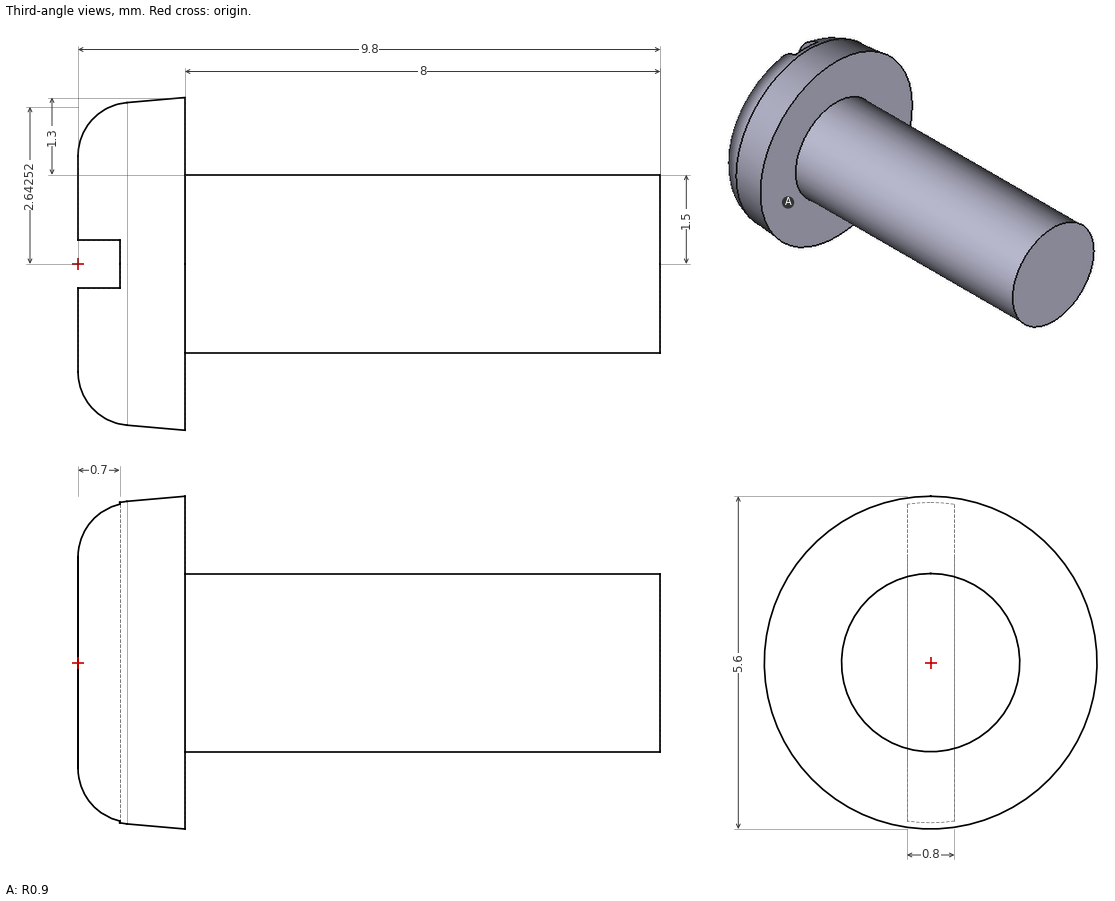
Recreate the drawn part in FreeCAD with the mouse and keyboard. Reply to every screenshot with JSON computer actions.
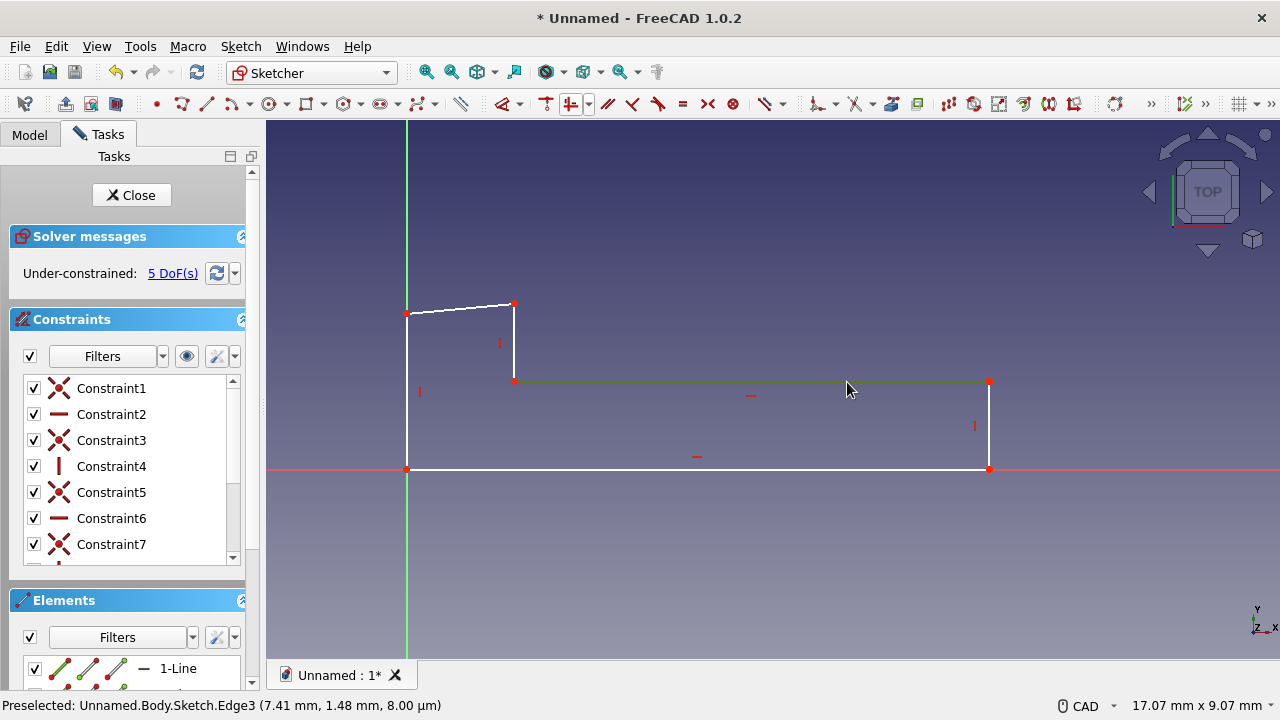
{"action": "left_click", "coordinate": [520, 104]}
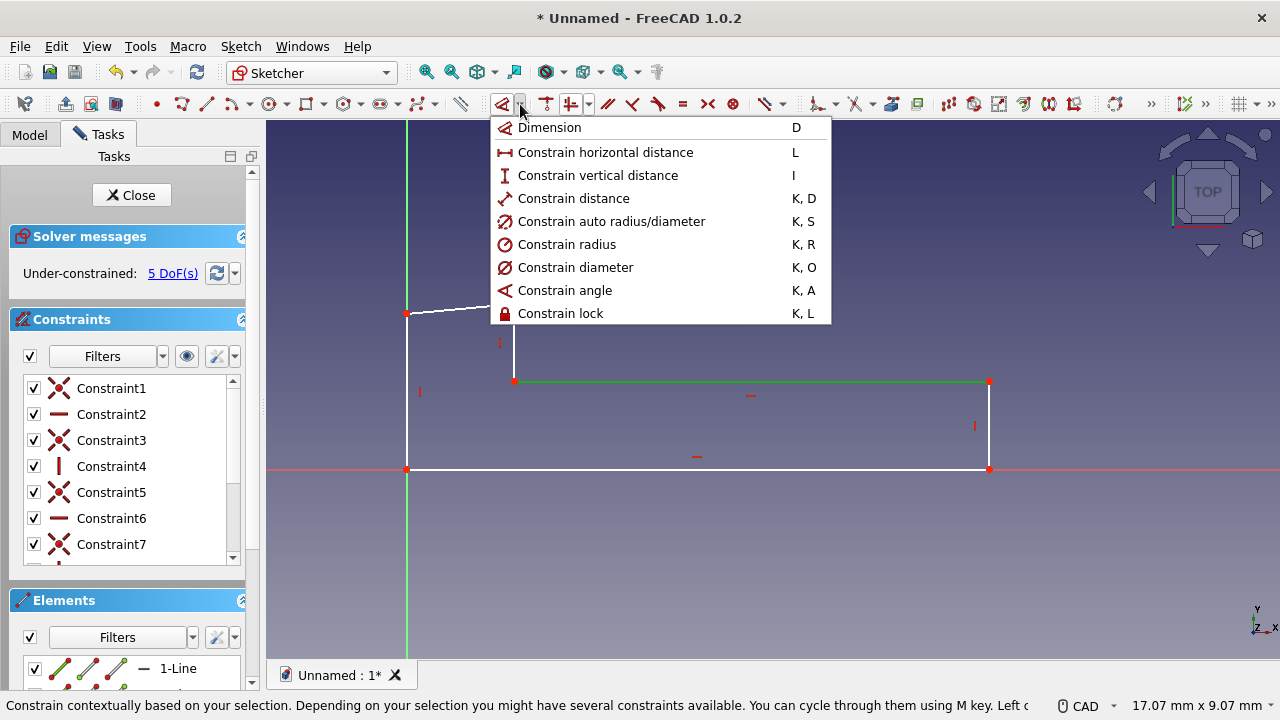
{"action": "left_click", "coordinate": [661, 152]}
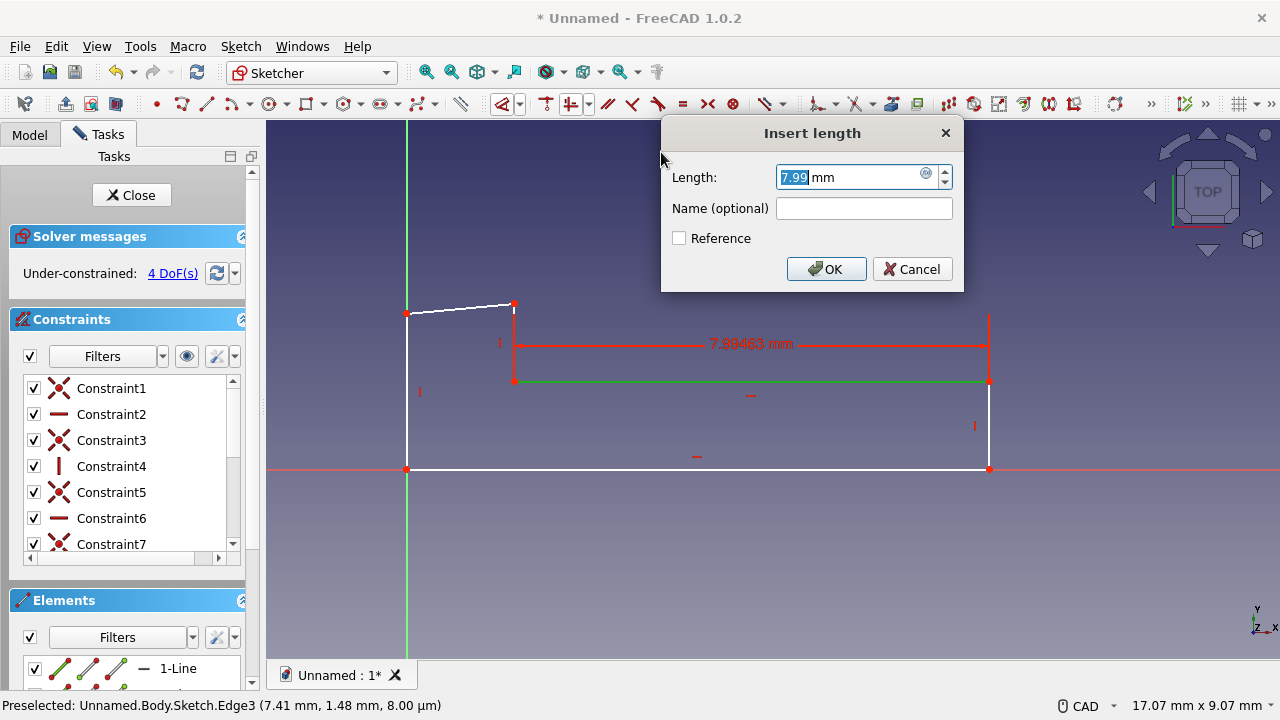
{"action": "type", "text": "8"}
{"action": "key", "text": "Return"}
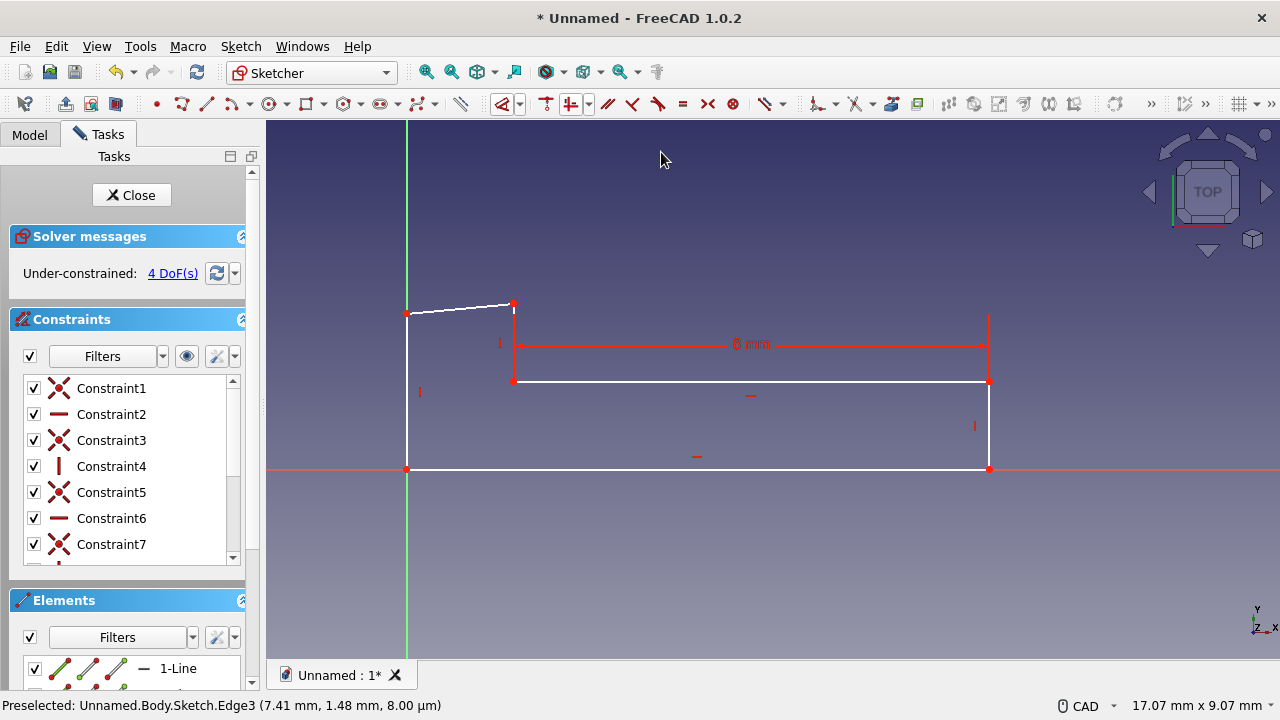
{"action": "left_click", "coordinate": [581, 470]}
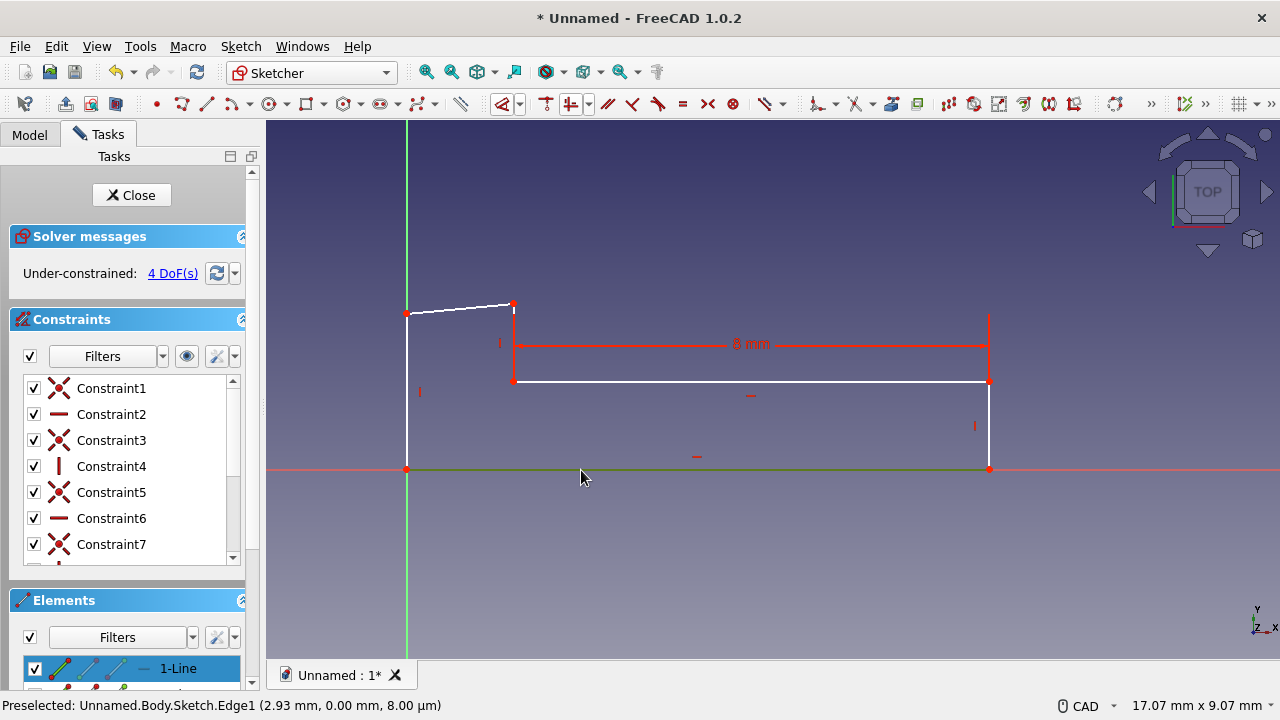
{"action": "key", "text": "l"}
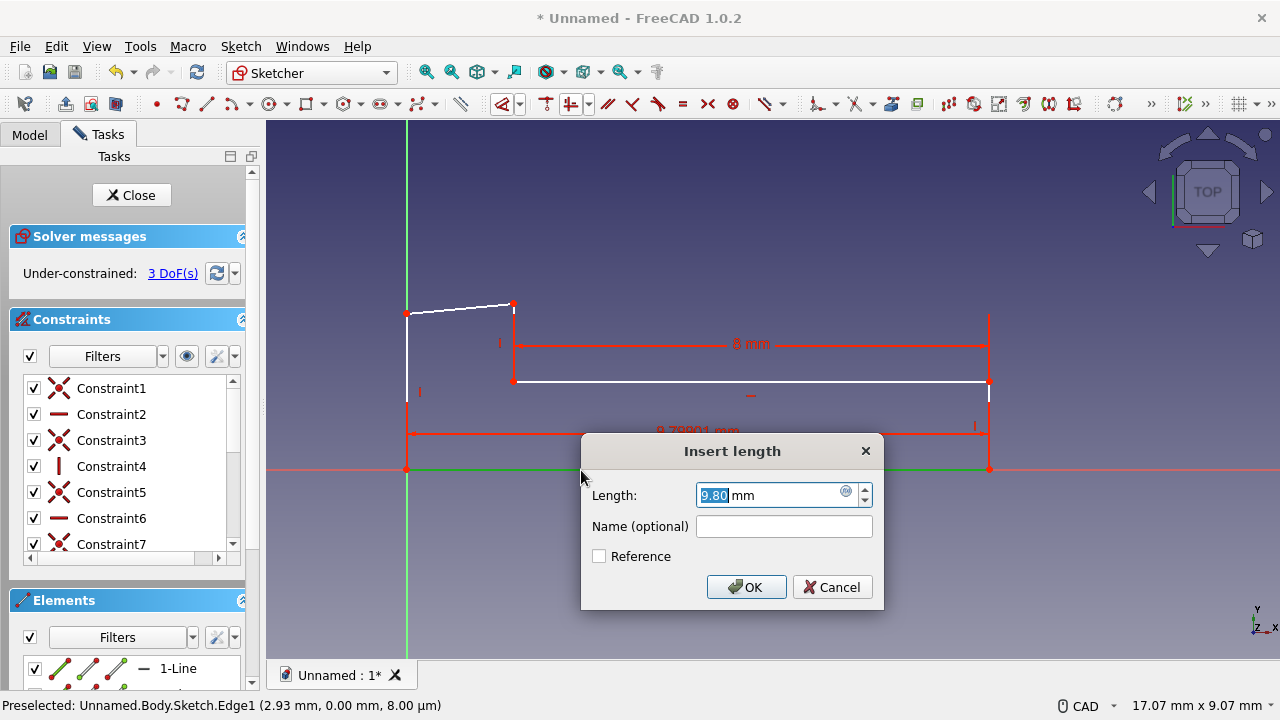
{"action": "type", "text": "9.8"}
{"action": "key", "text": "Return"}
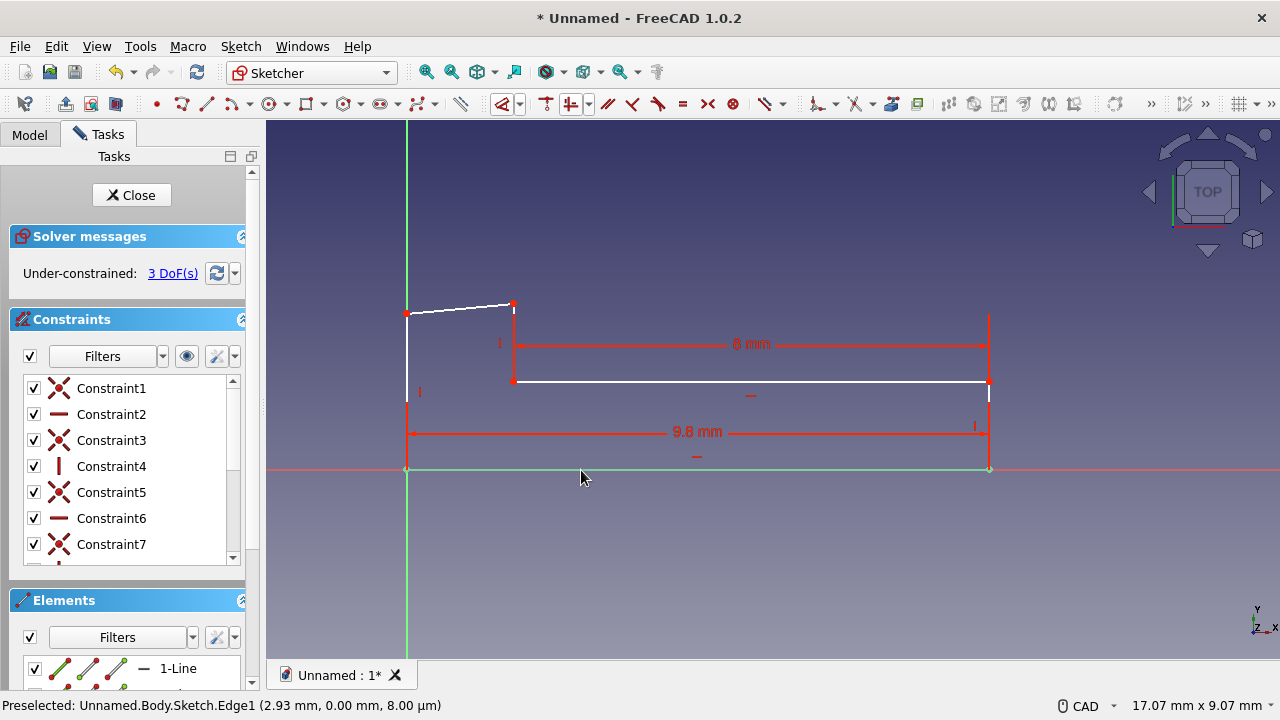
{"action": "left_click", "coordinate": [989, 443]}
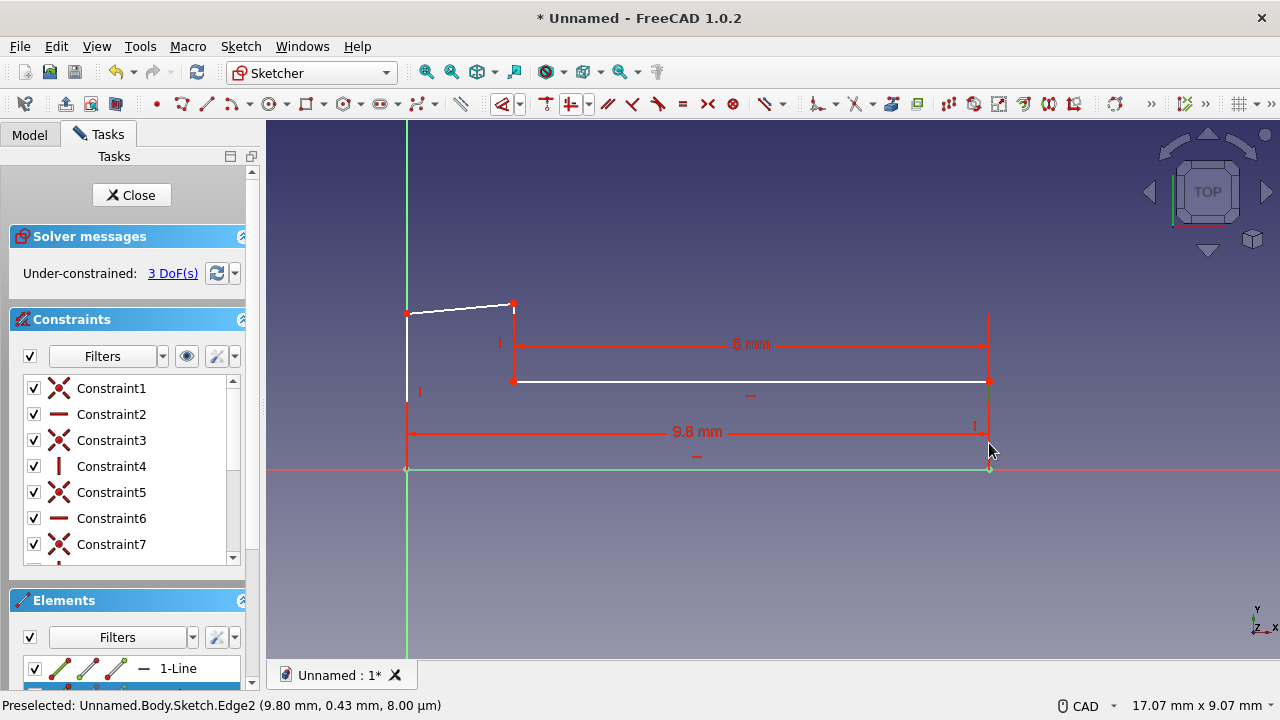
{"action": "left_click", "coordinate": [520, 104]}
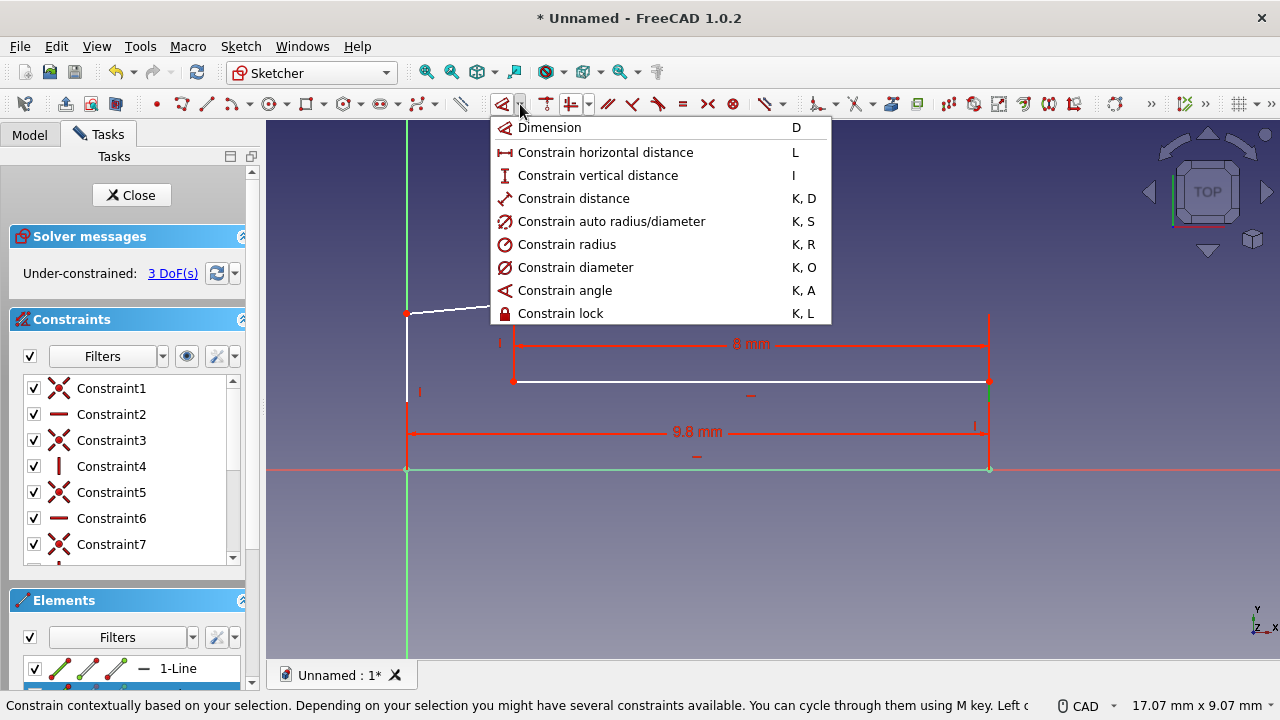
{"action": "left_click", "coordinate": [661, 176]}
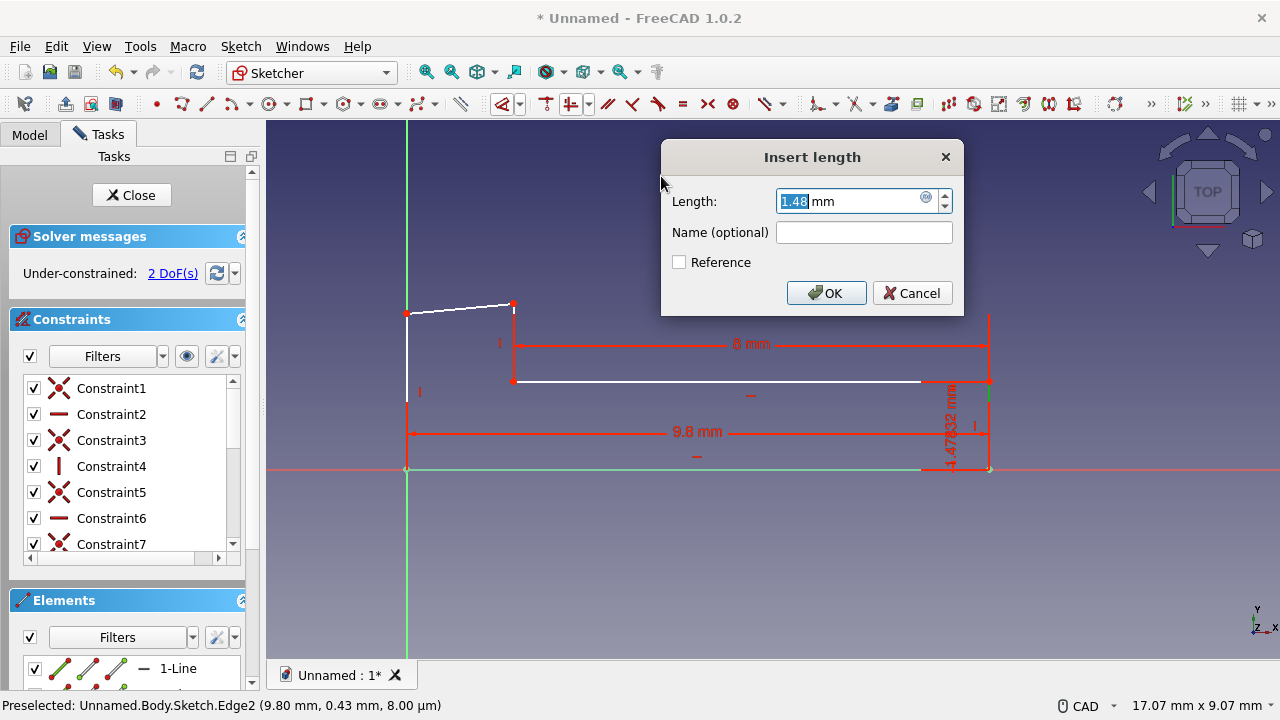
{"action": "type", "text": "1.5"}
{"action": "key", "text": "Return"}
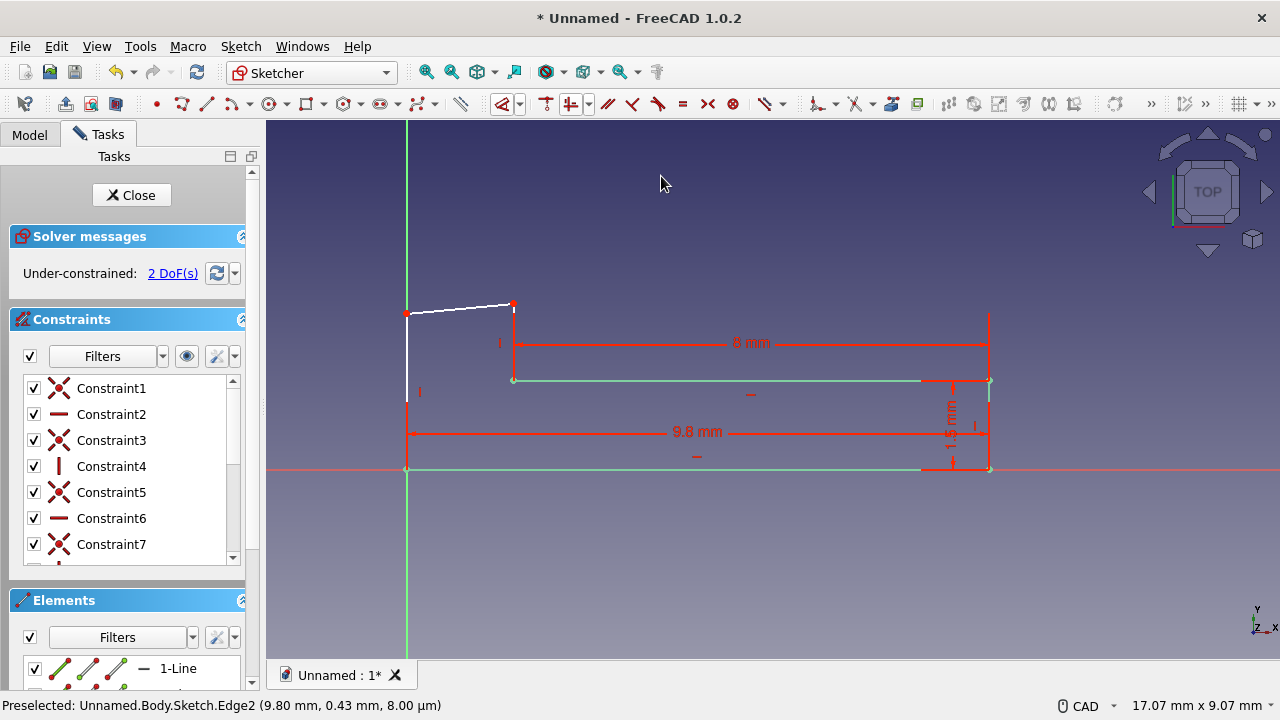
{"action": "left_click", "coordinate": [514, 358]}